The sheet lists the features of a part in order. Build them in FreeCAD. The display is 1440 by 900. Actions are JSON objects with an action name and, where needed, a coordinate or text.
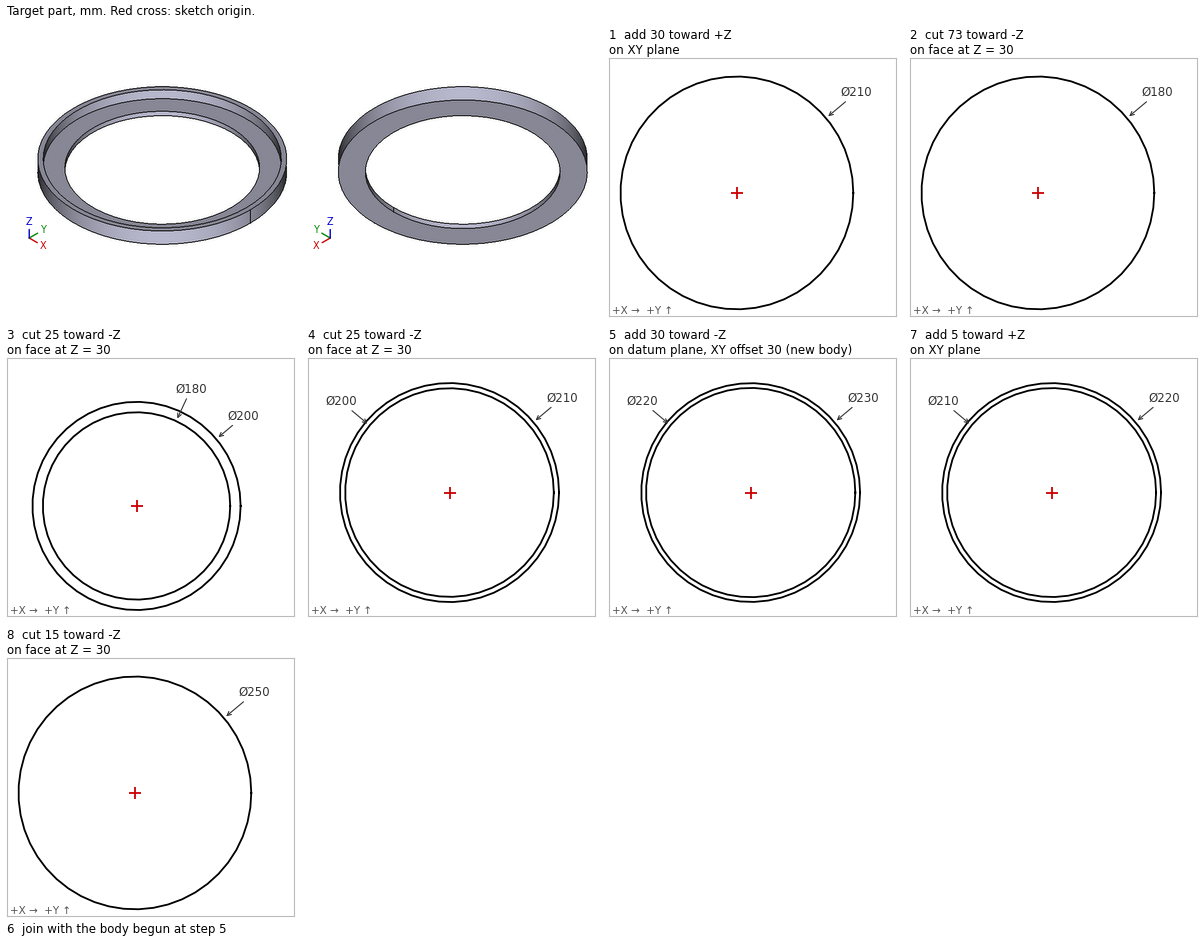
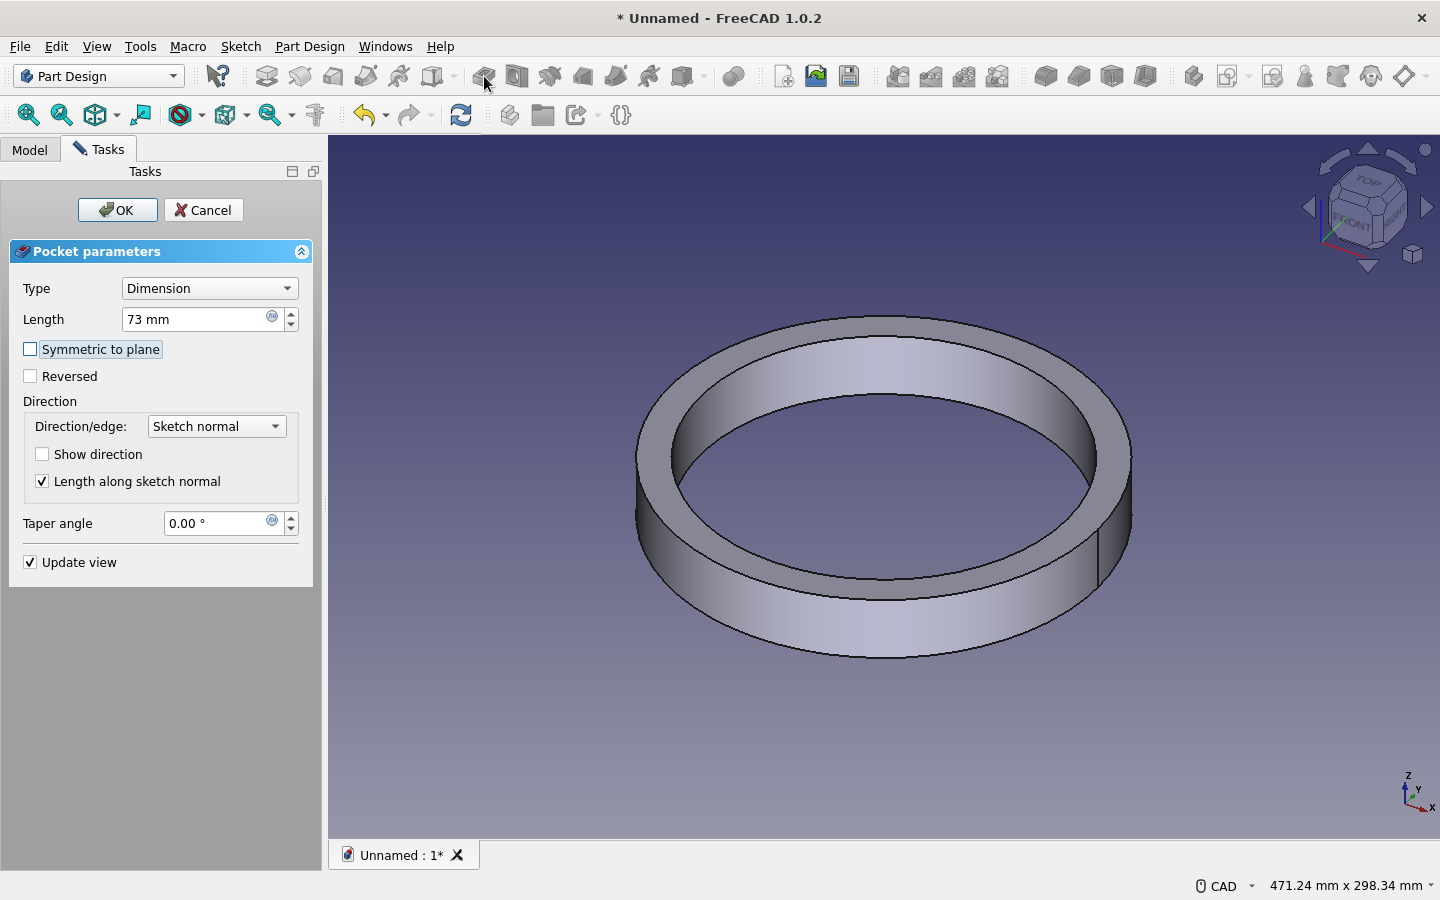
{"action": "left_click", "coordinate": [118, 210]}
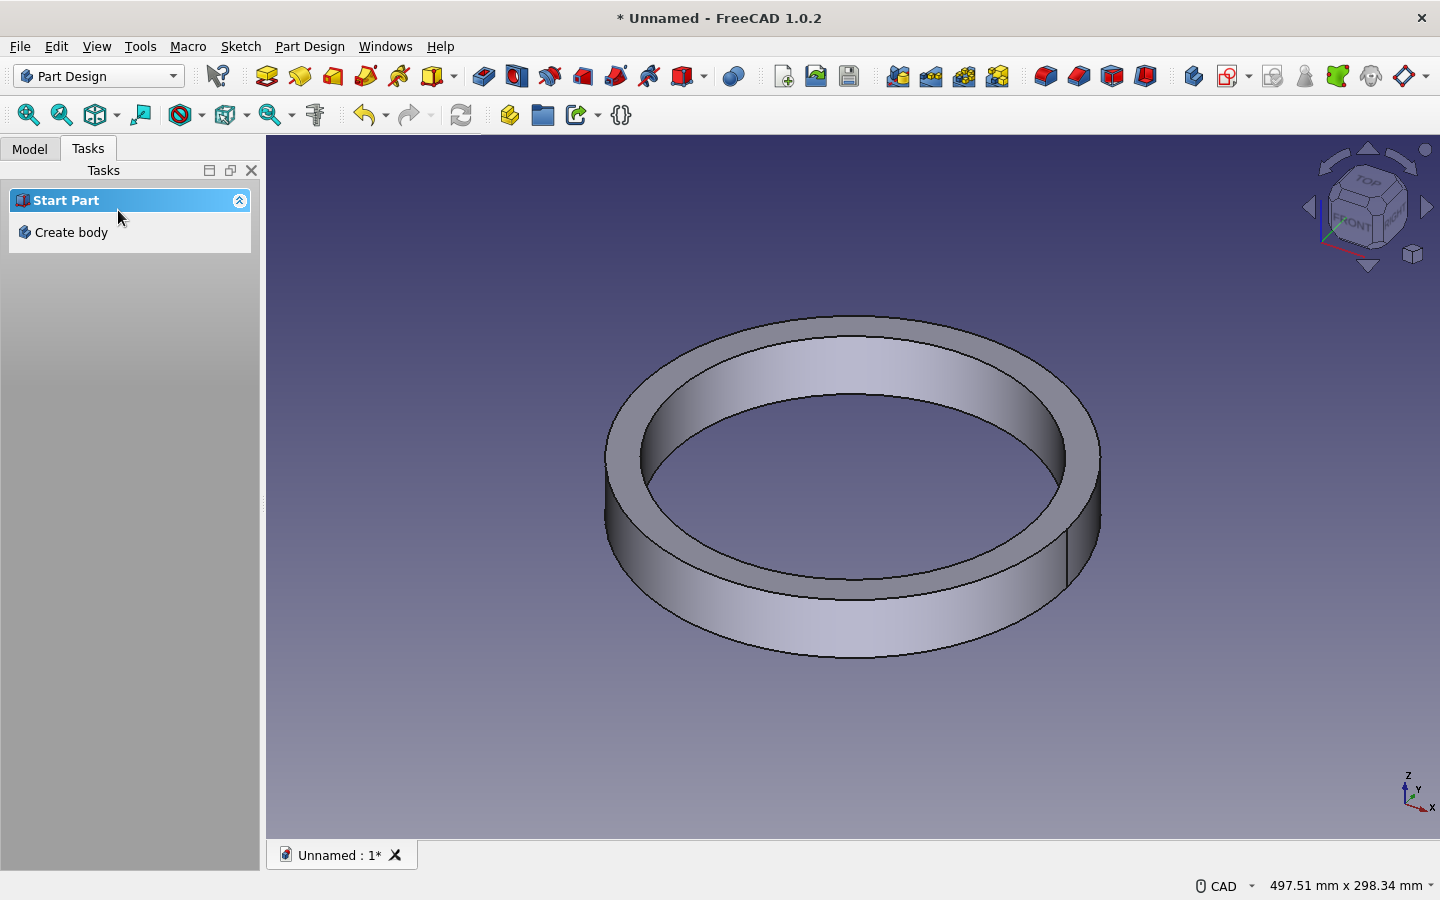
{"action": "left_click", "coordinate": [1072, 483]}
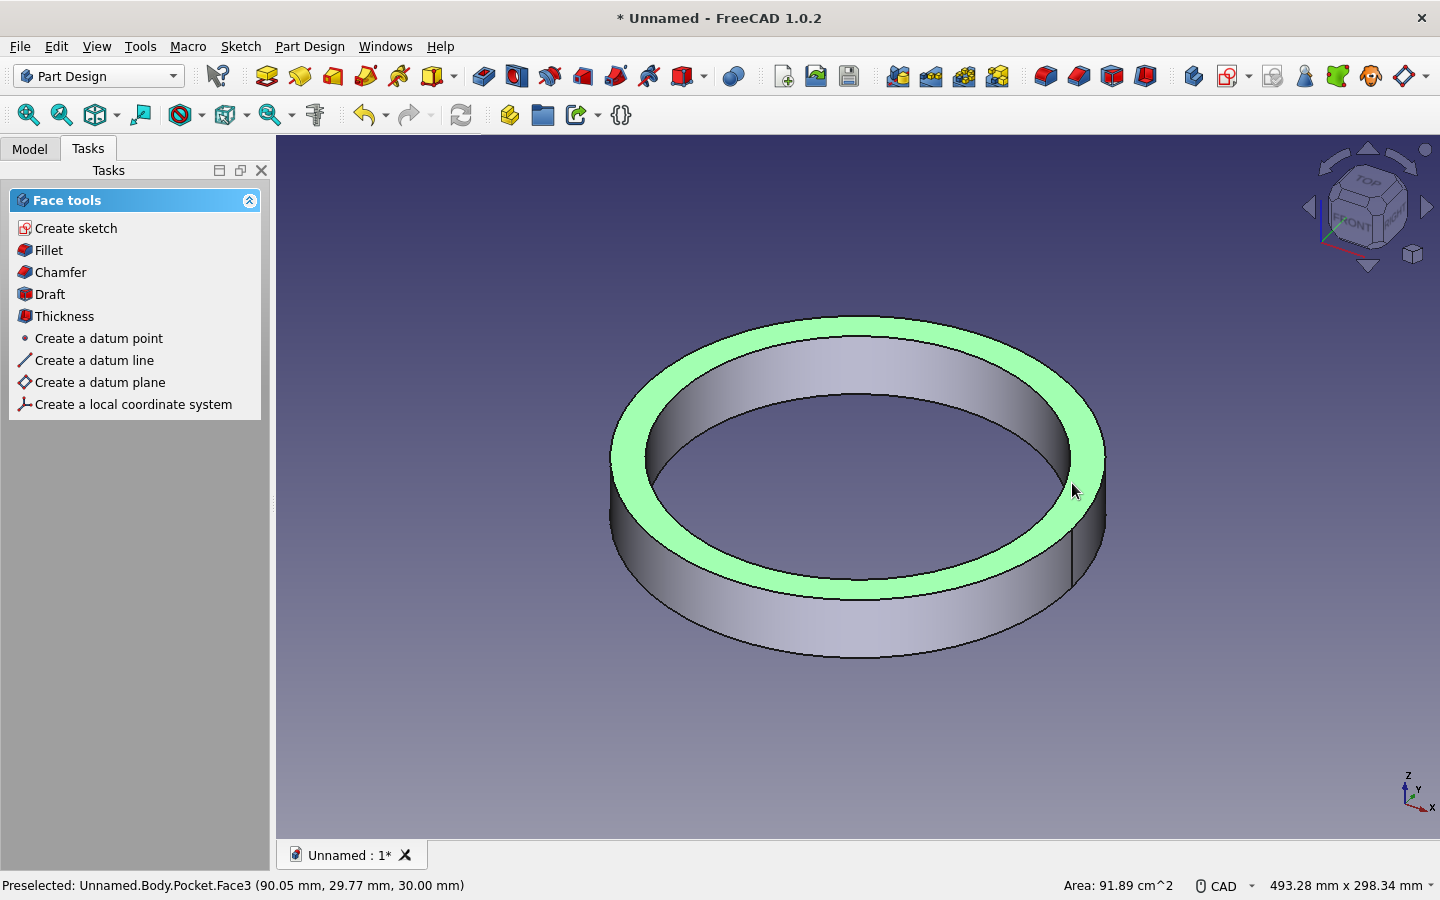
{"action": "left_click", "coordinate": [1226, 76]}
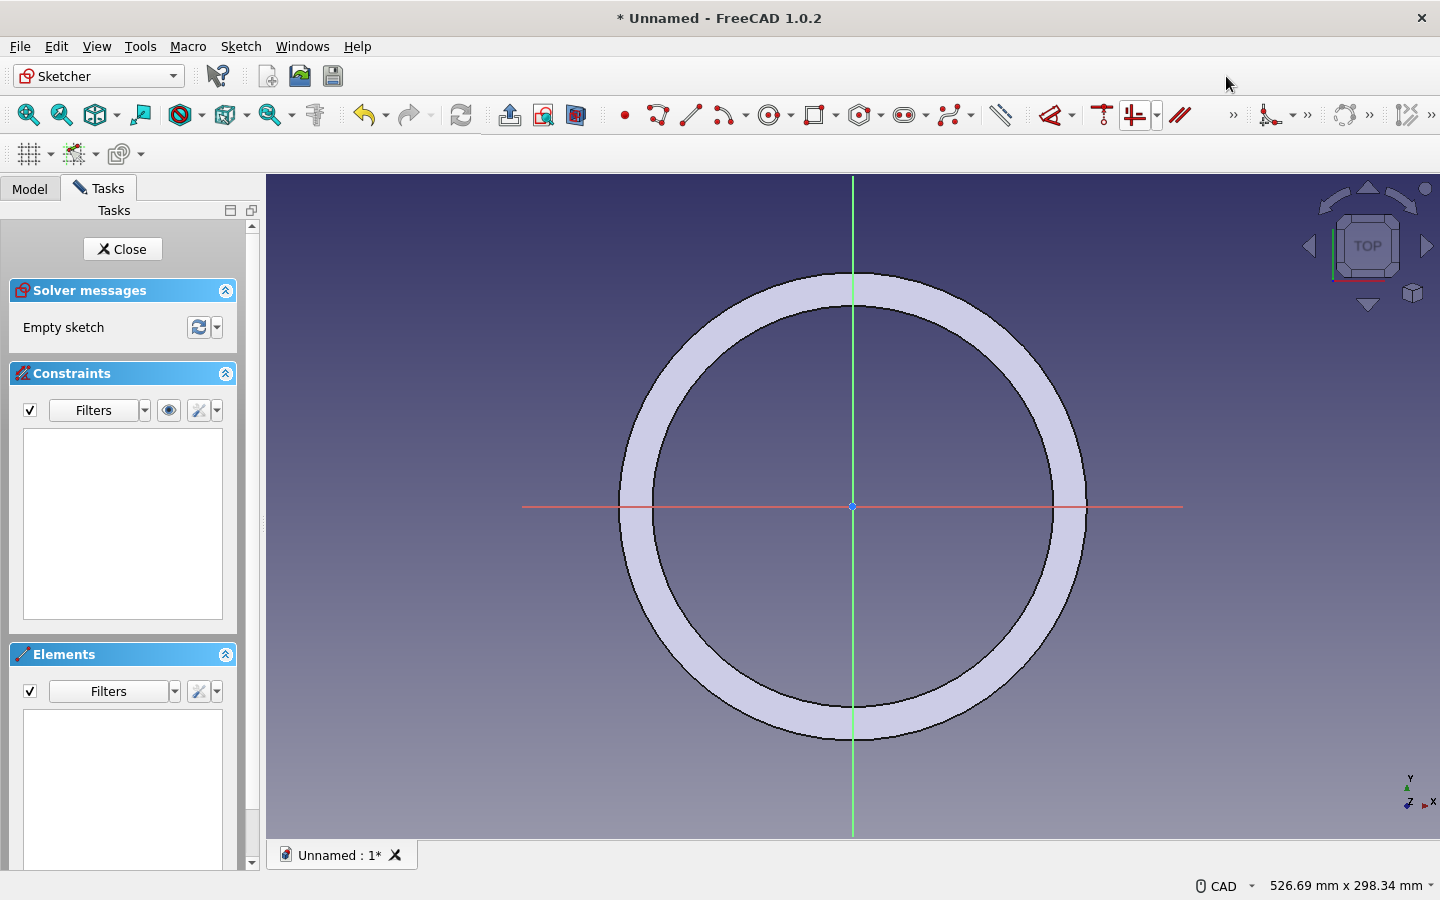
{"action": "left_click", "coordinate": [768, 116]}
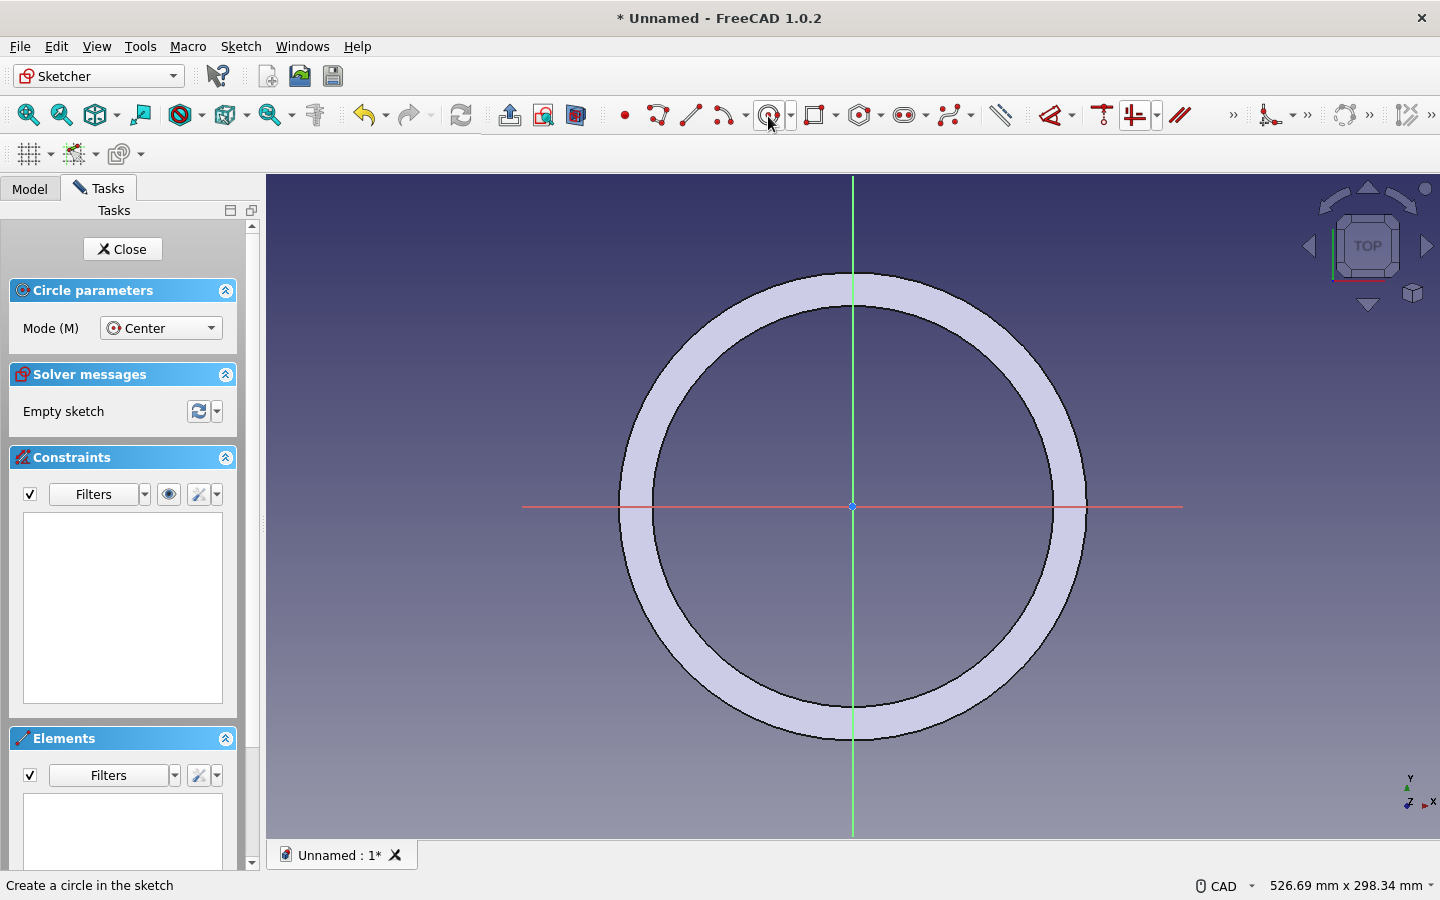
{"action": "left_click", "coordinate": [853, 506]}
{"action": "mouse_move", "coordinate": [1010, 349]}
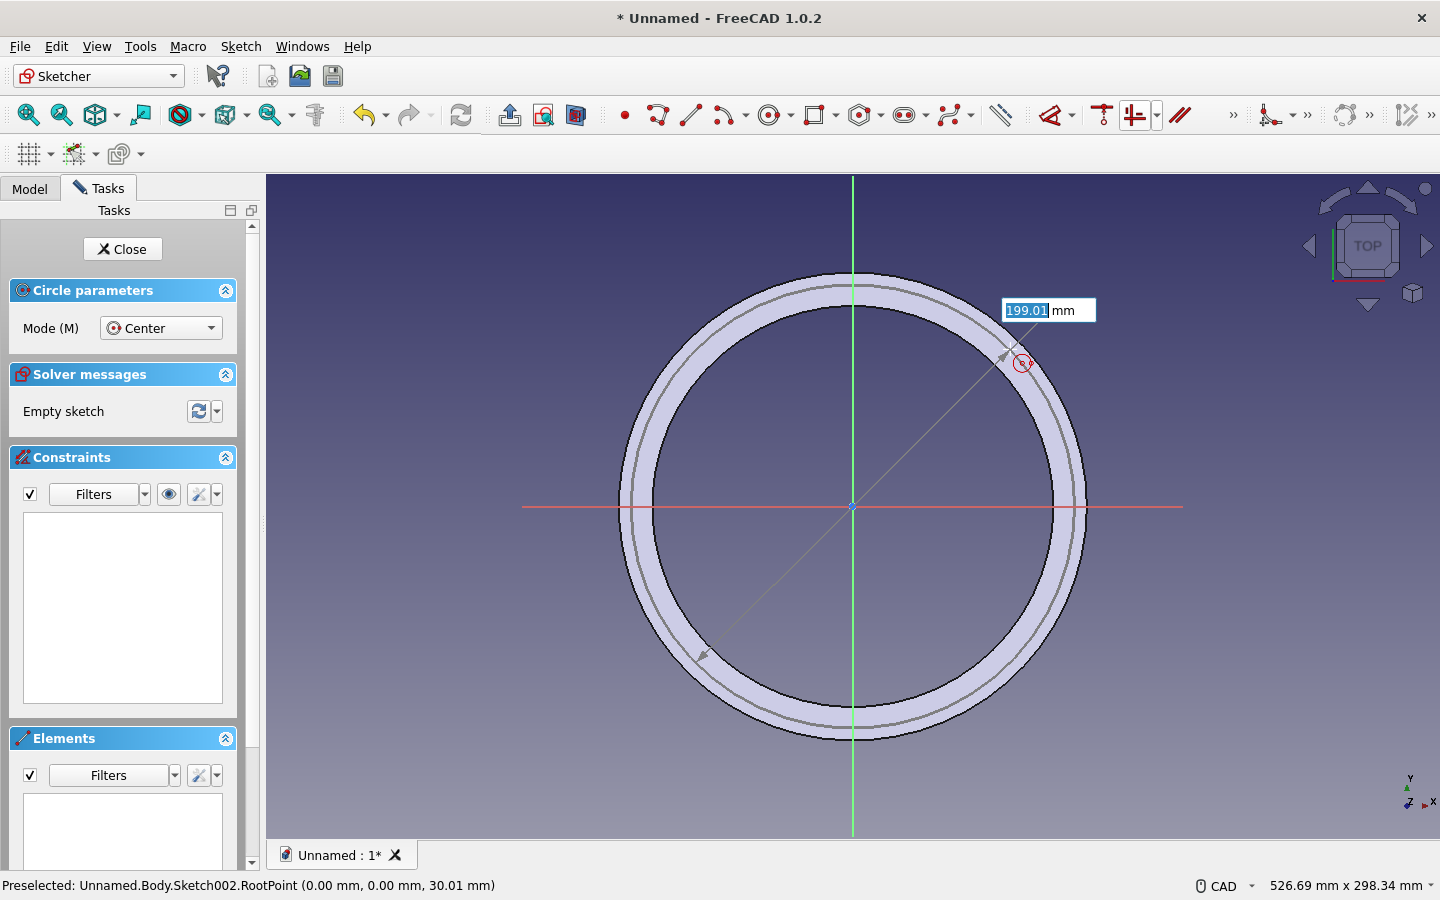
{"action": "type", "text": "200"}
{"action": "key", "text": "Return"}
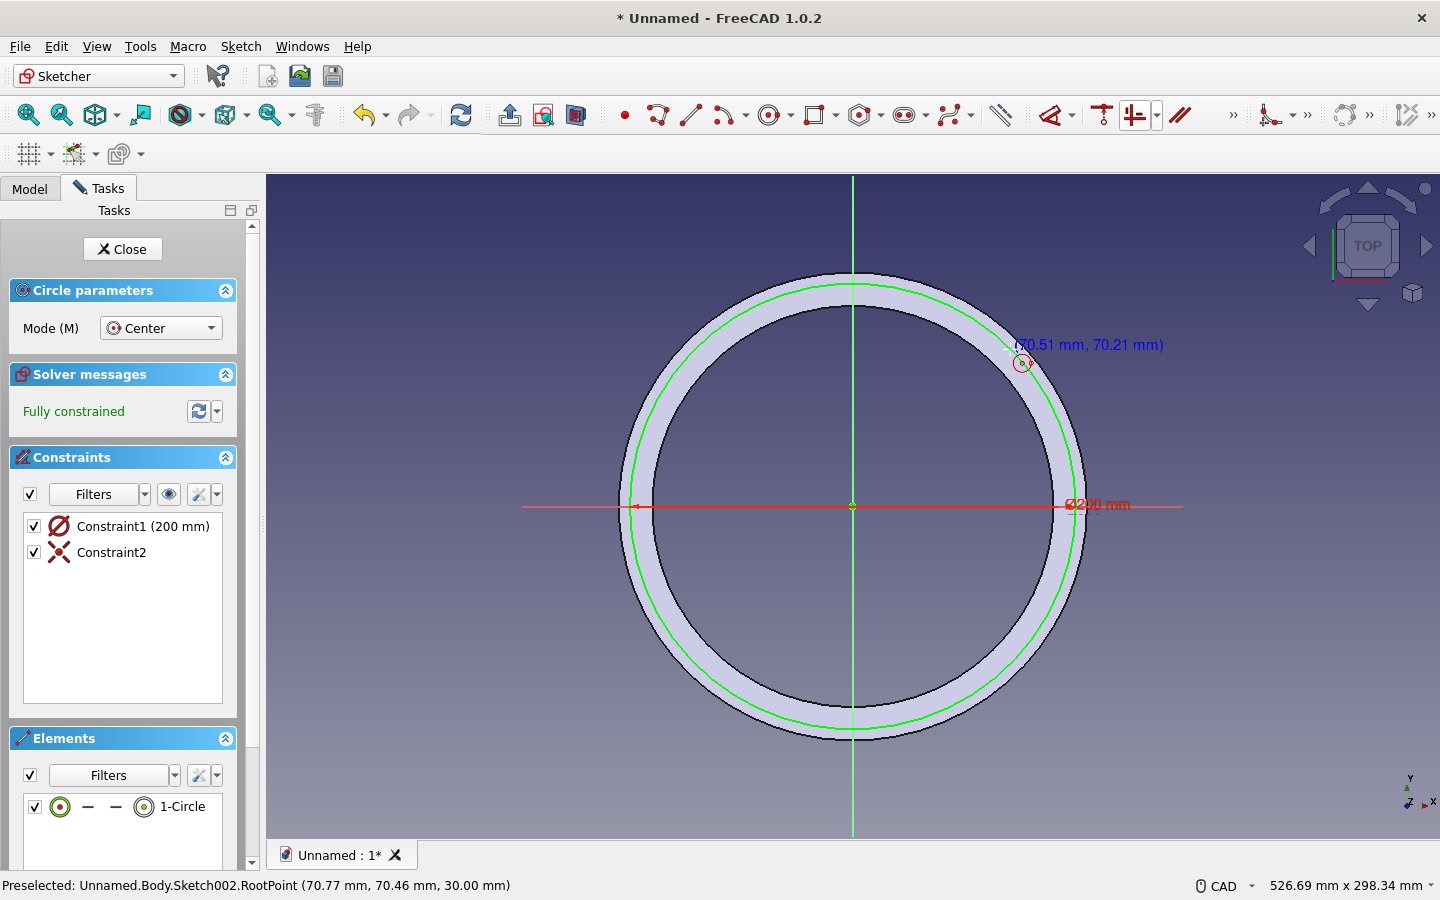
{"action": "left_click", "coordinate": [853, 506]}
{"action": "mouse_move", "coordinate": [995, 365]}